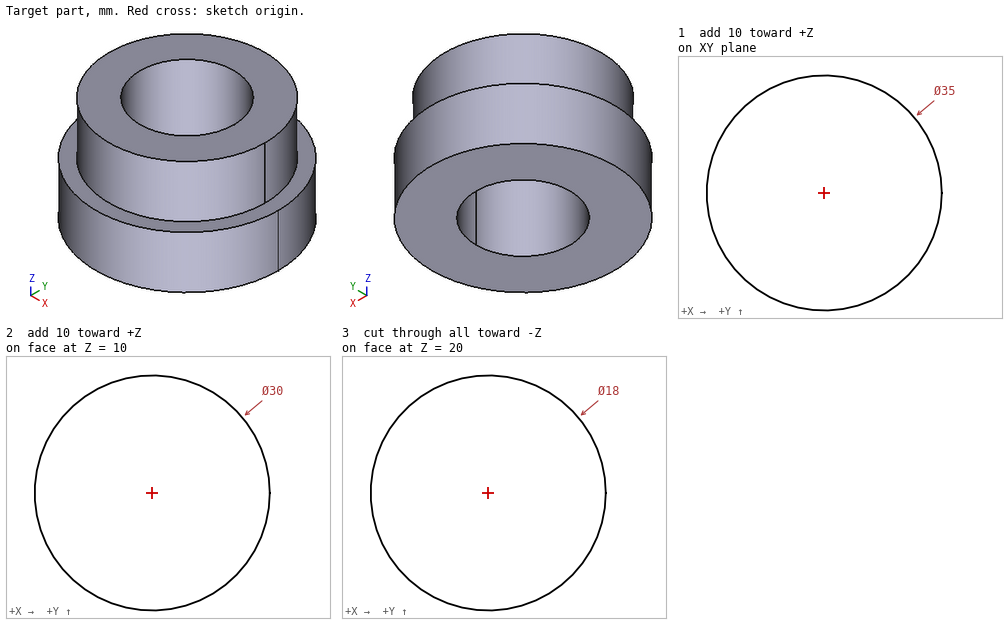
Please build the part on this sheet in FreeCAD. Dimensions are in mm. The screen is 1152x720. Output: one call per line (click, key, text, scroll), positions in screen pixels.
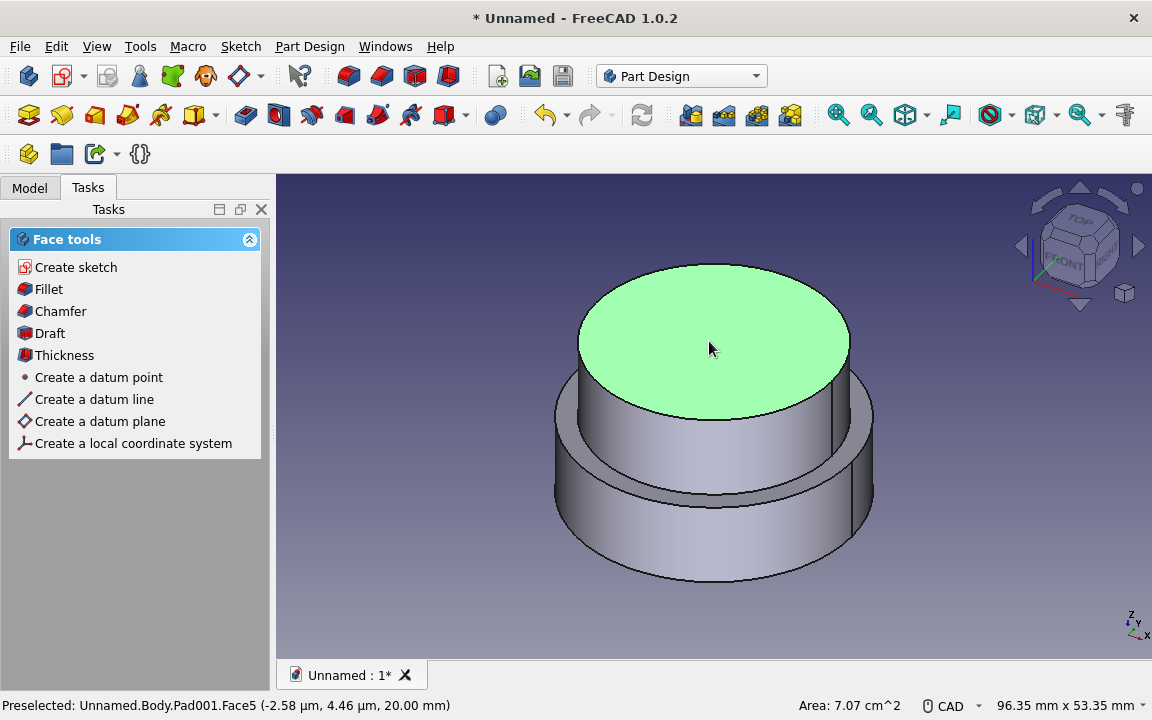
click(62, 76)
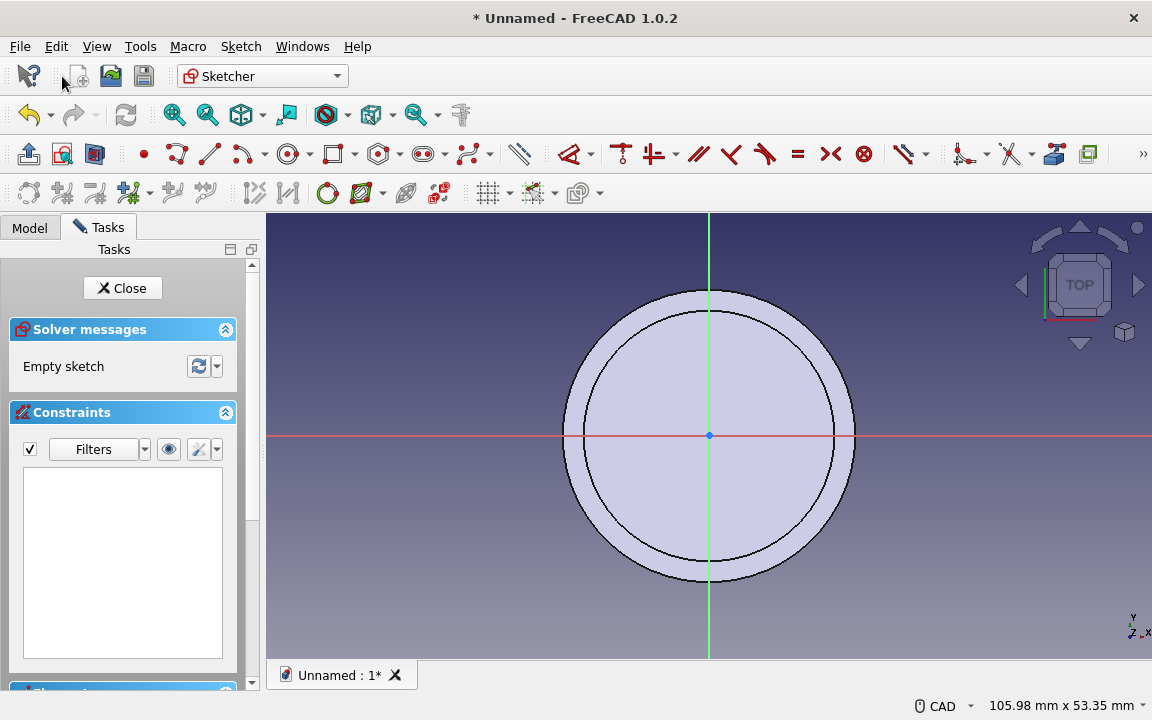
scroll(792, 436, up, 3)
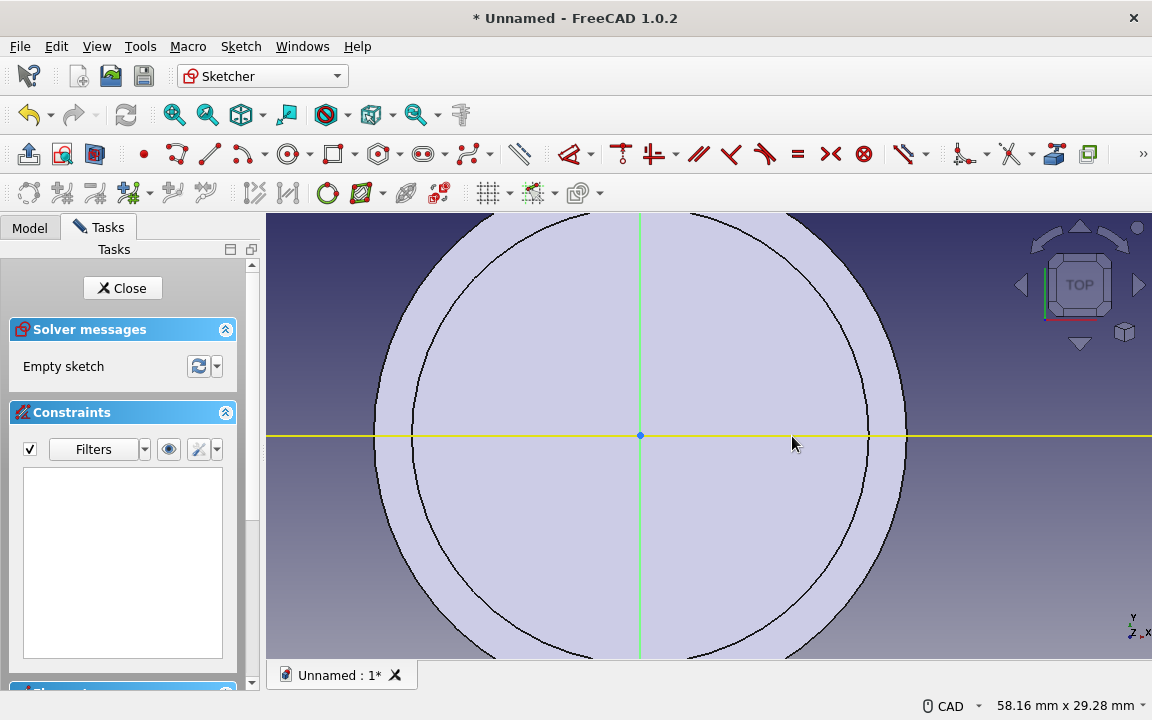
click(288, 154)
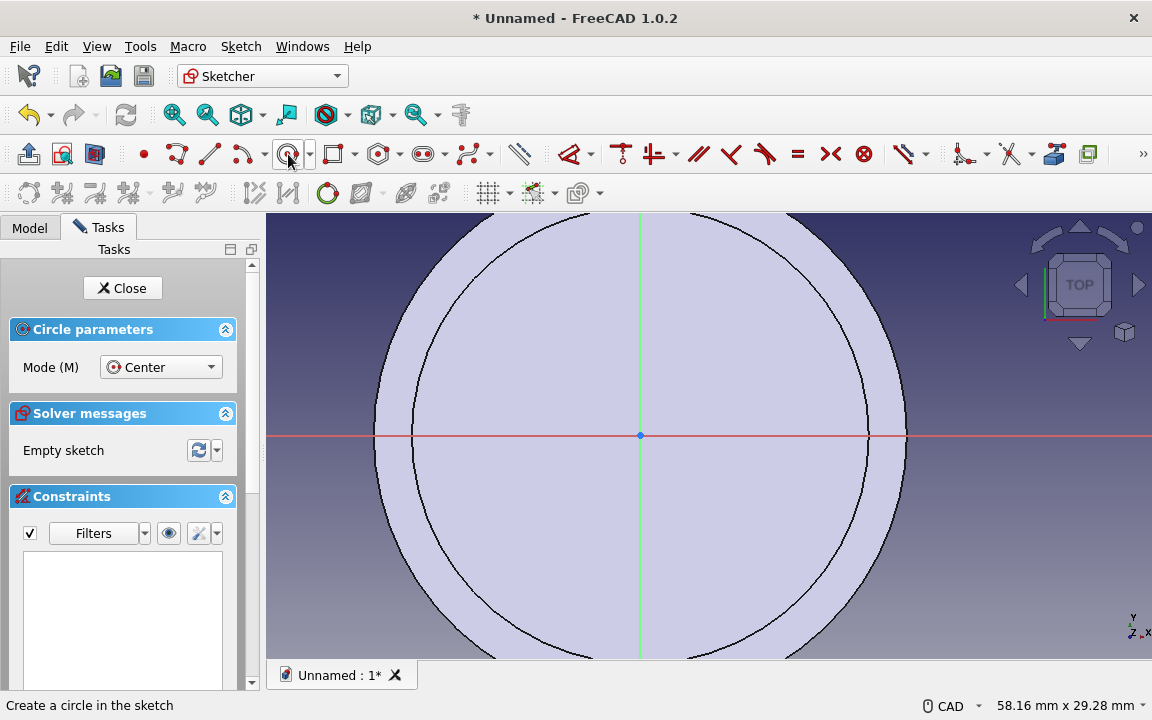
click(640, 436)
move(737, 339)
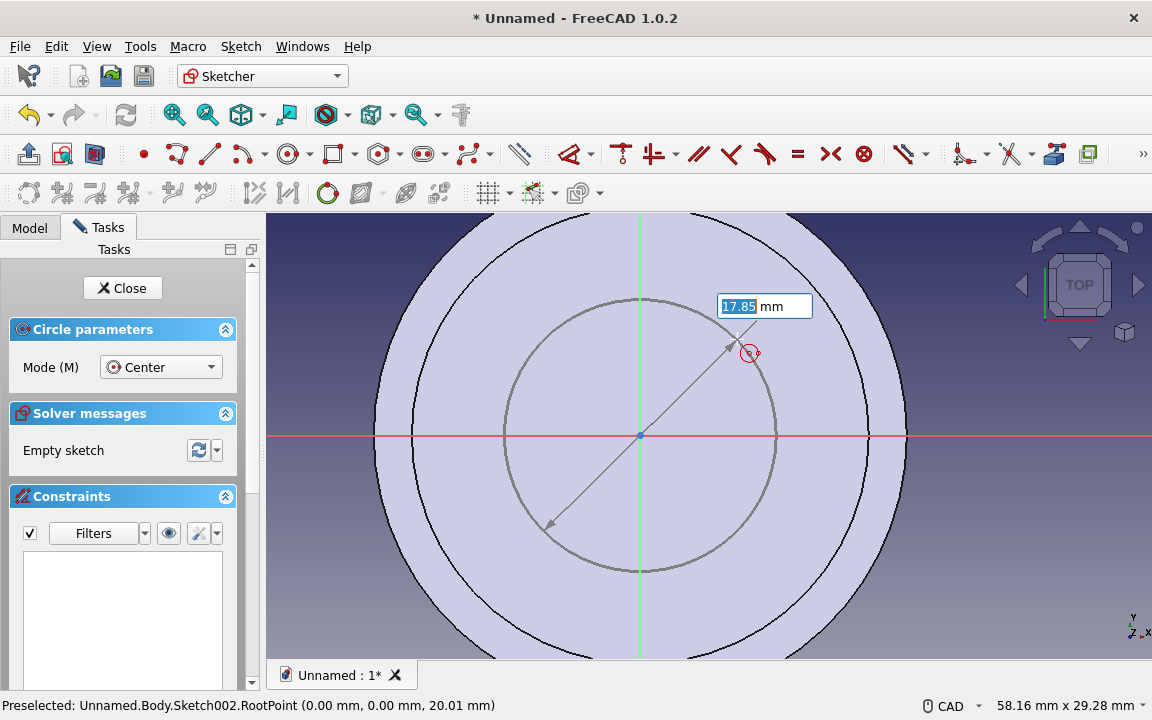
text(18)
key(Return)
key(Escape)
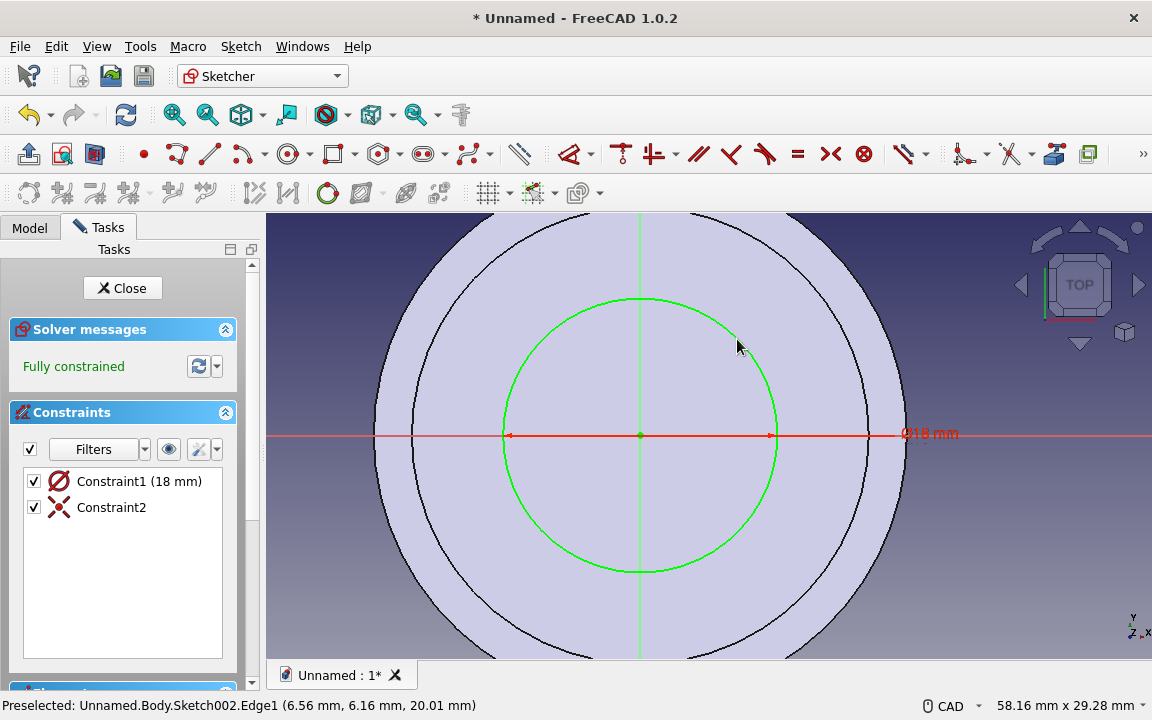
click(123, 288)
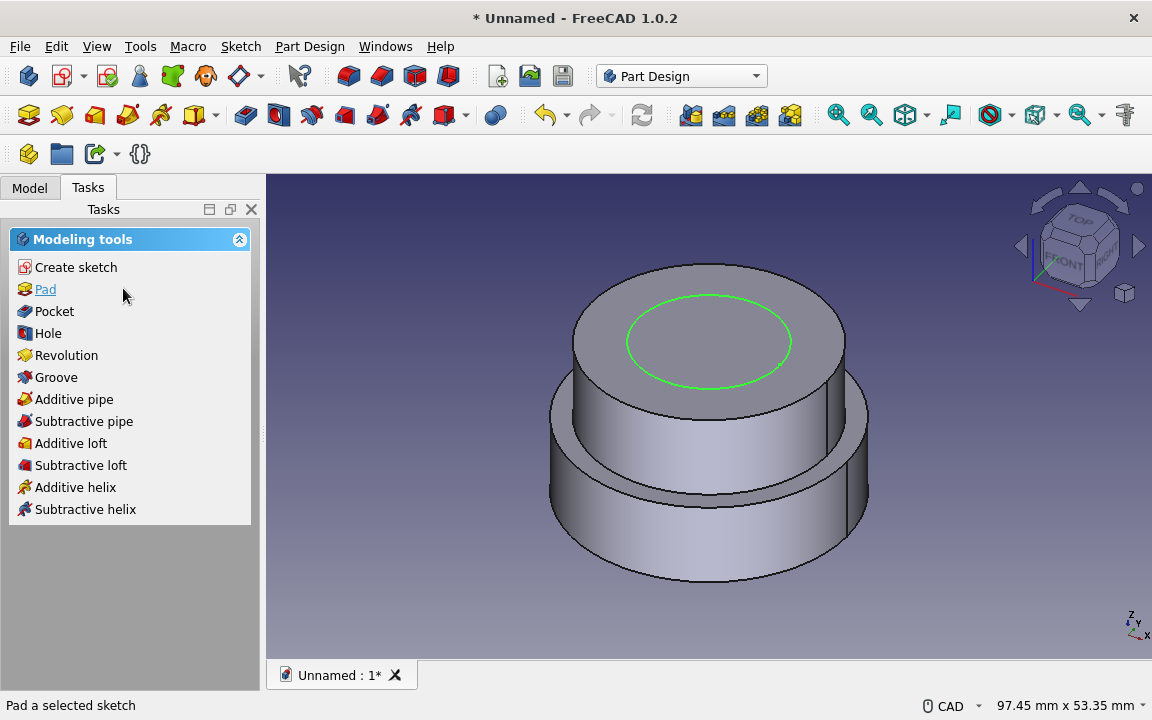
click(246, 116)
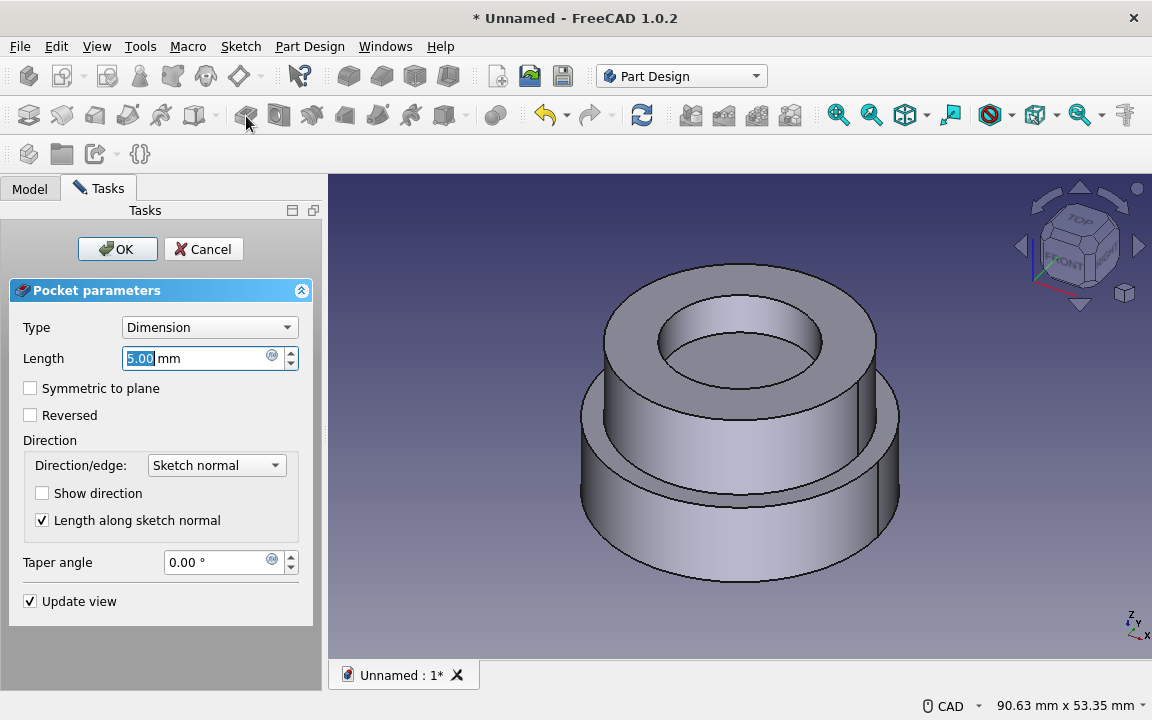
click(210, 328)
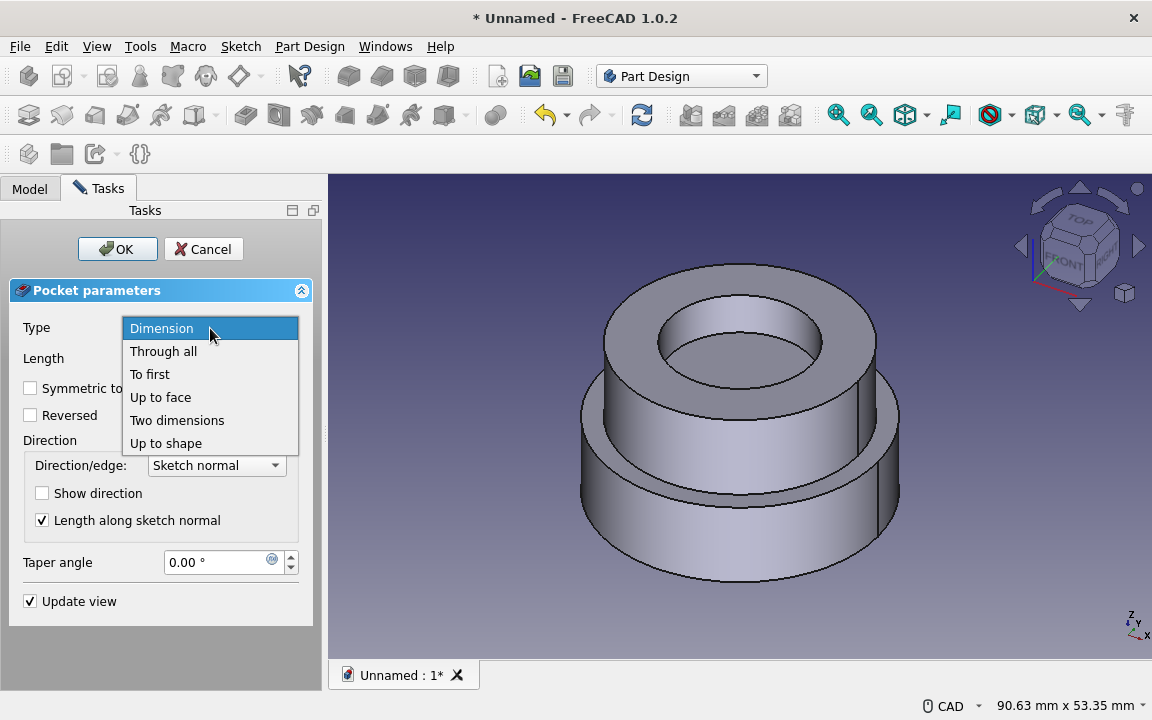
click(208, 352)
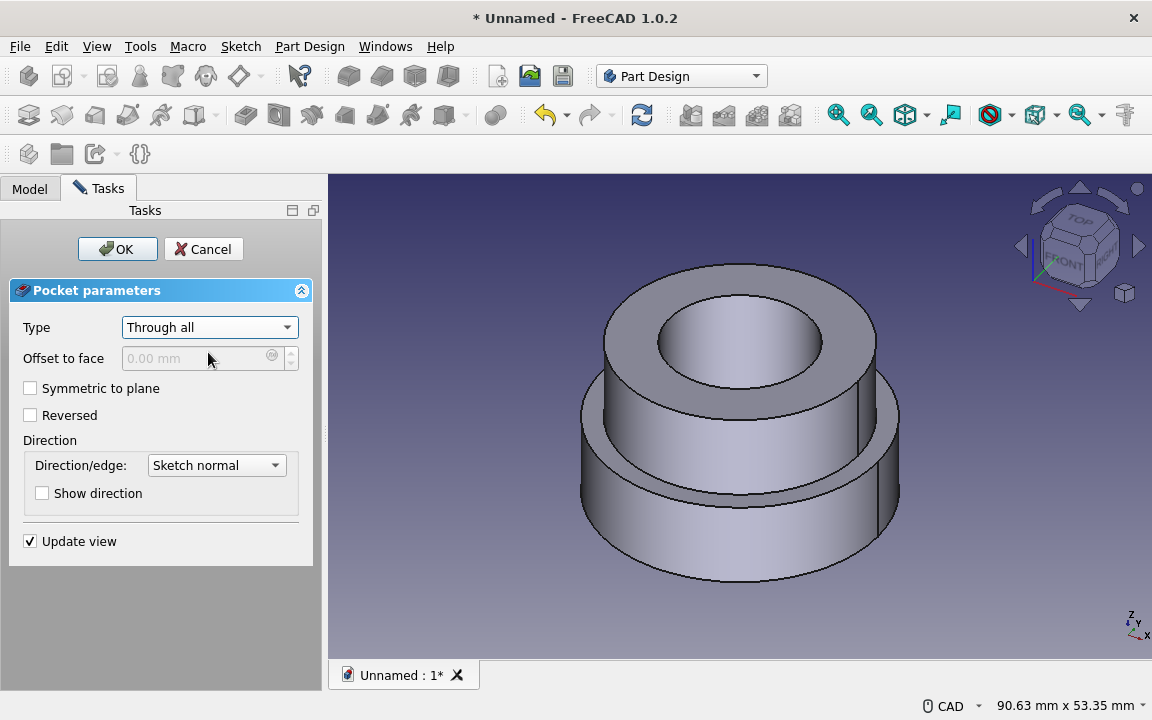
click(118, 249)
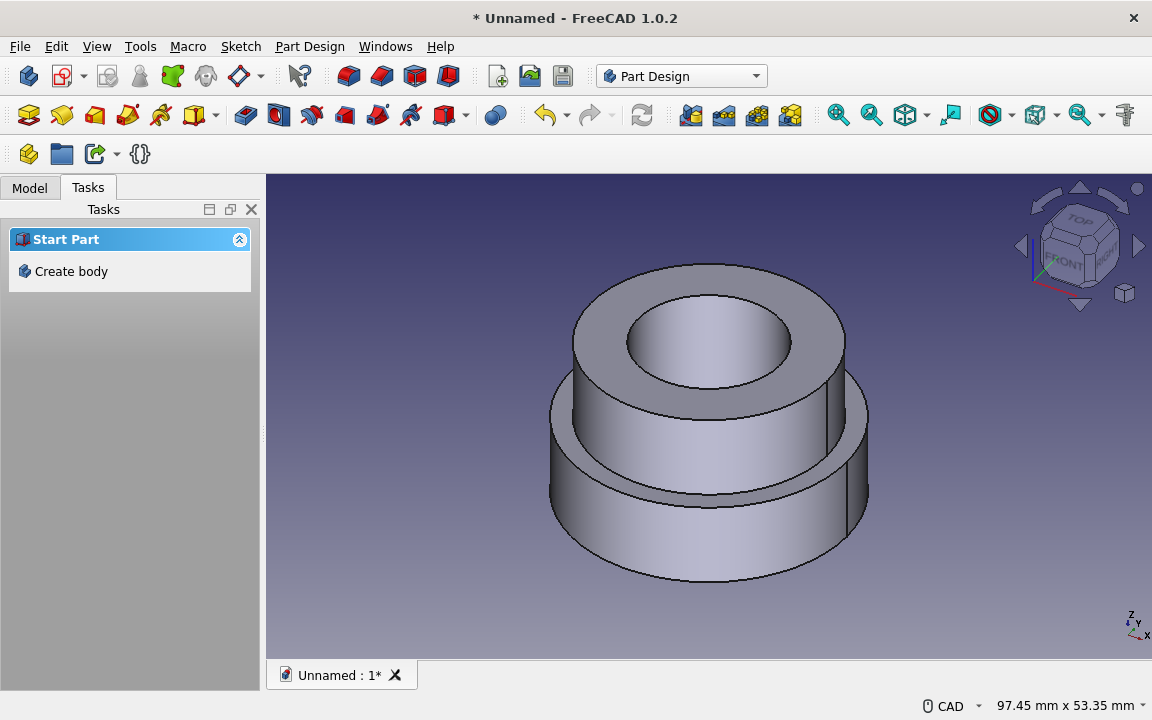
key(0)